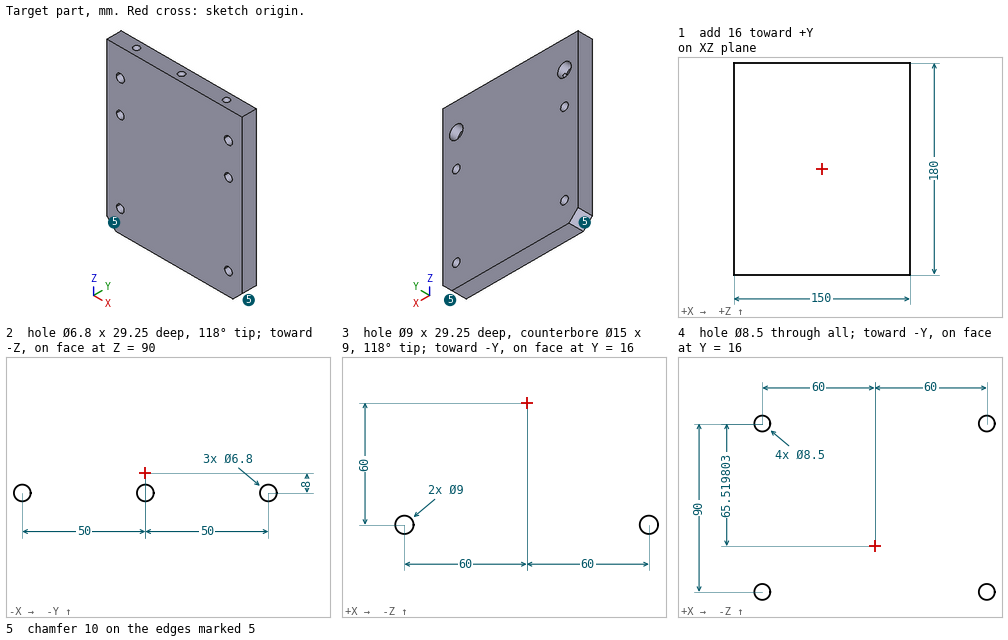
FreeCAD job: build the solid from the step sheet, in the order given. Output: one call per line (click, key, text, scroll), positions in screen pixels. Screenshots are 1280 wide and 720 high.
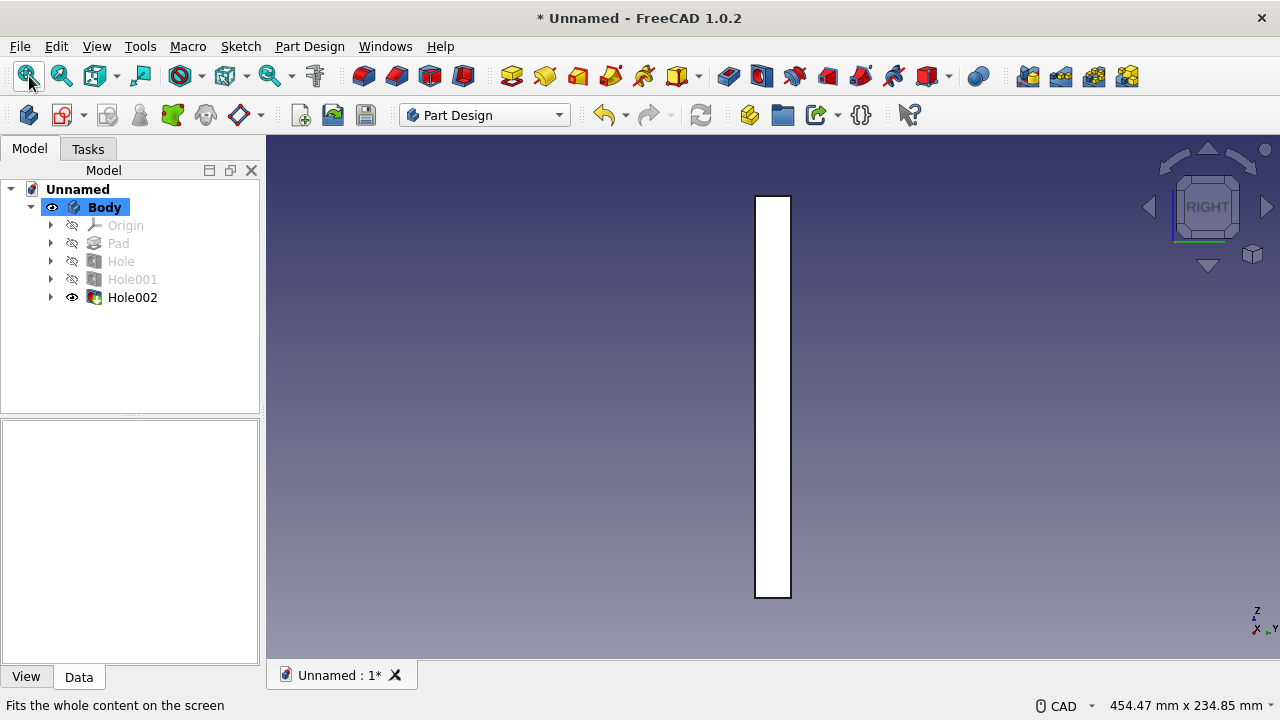
click(773, 597)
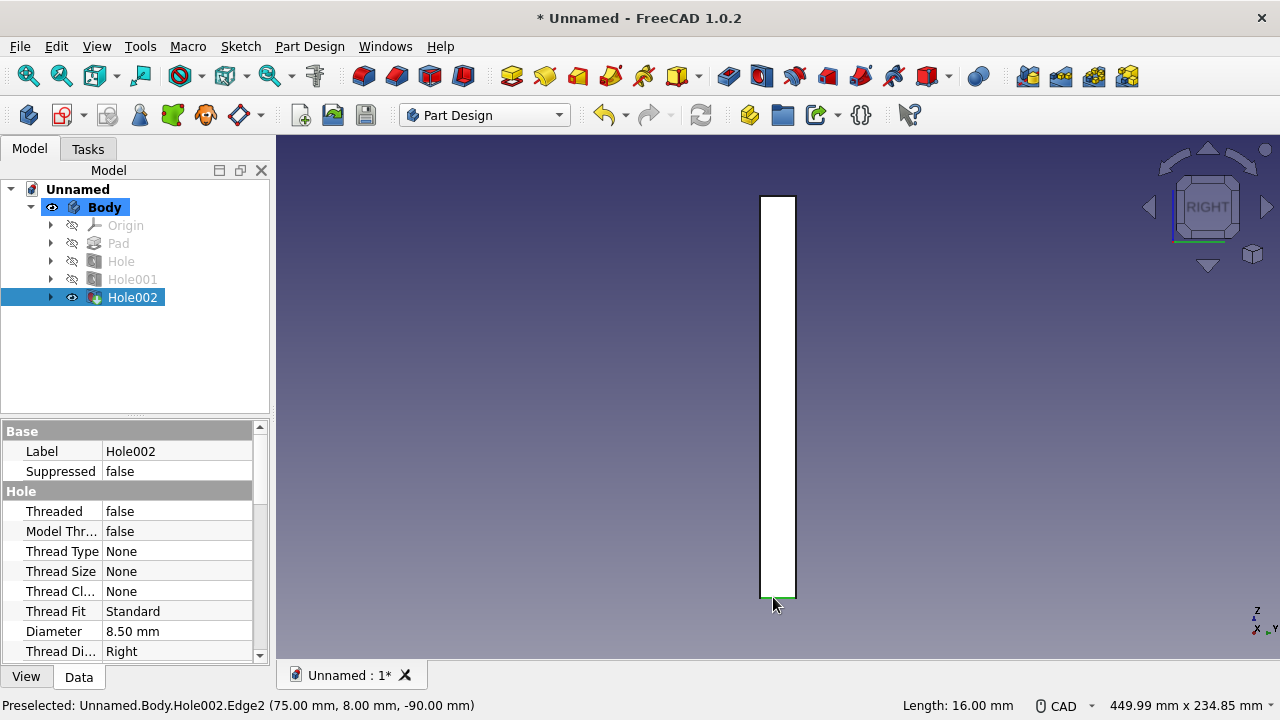
key(5)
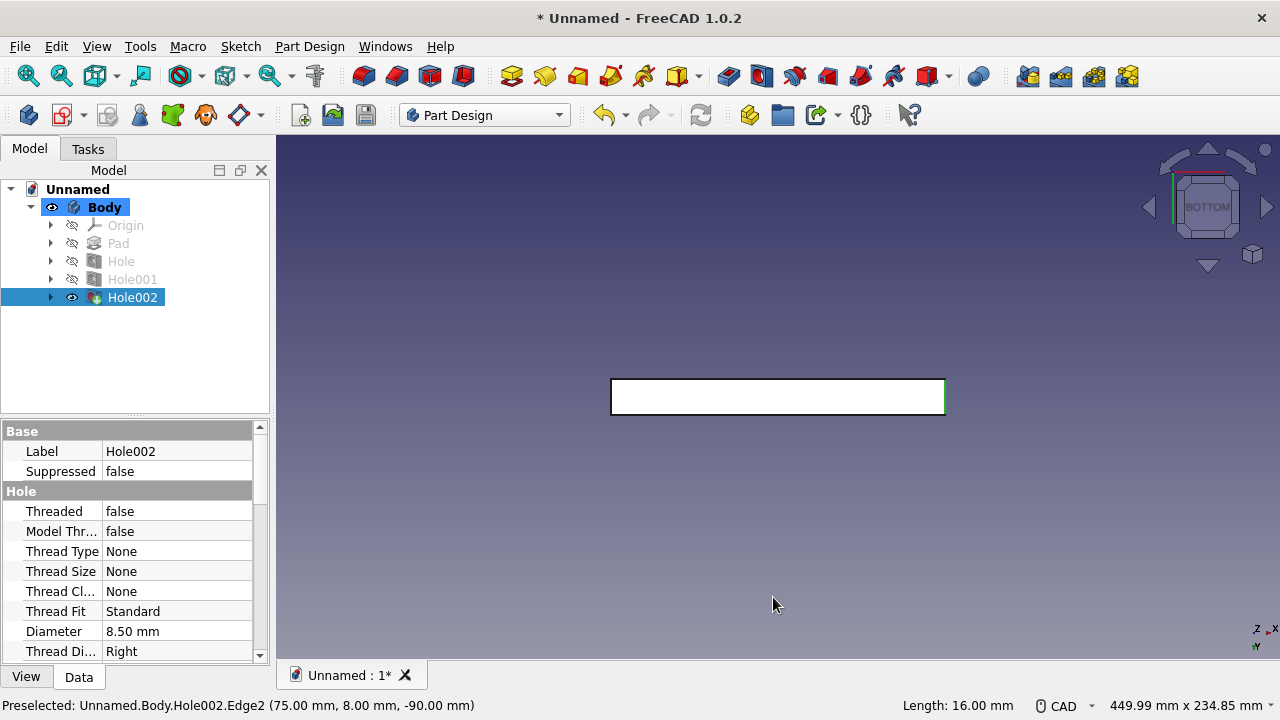
click(29, 76)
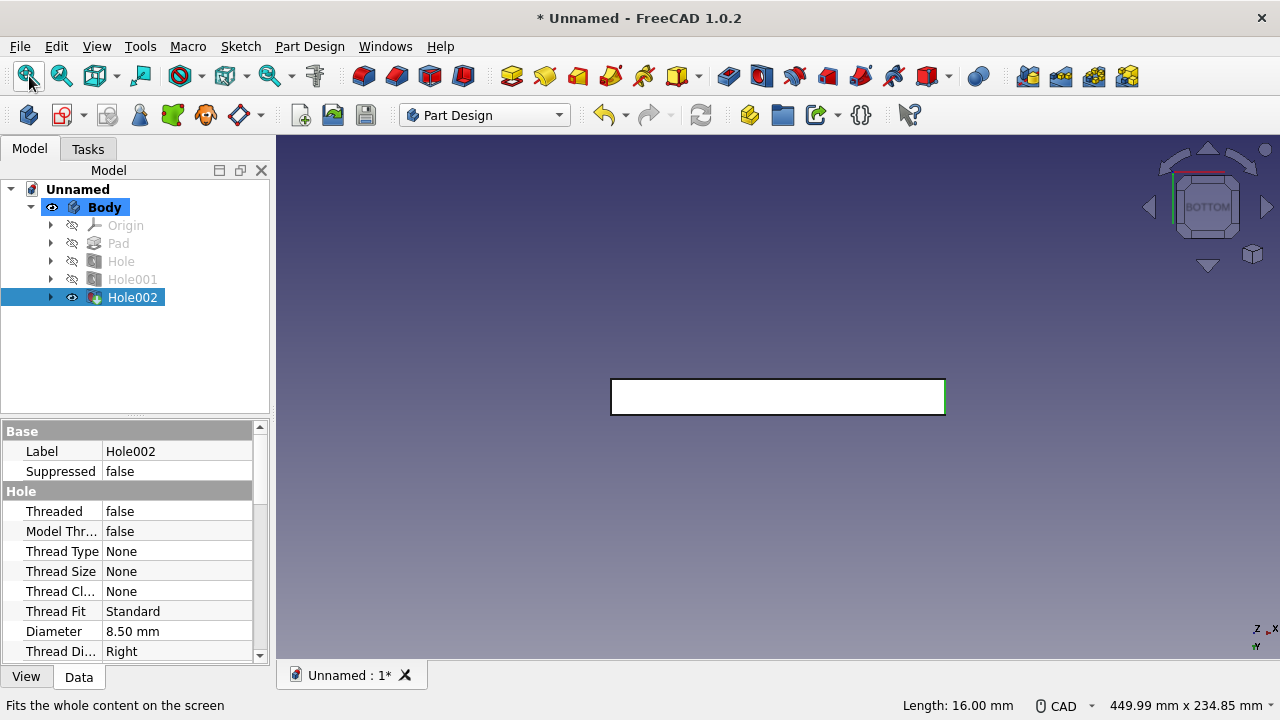
click(611, 396, ctrl)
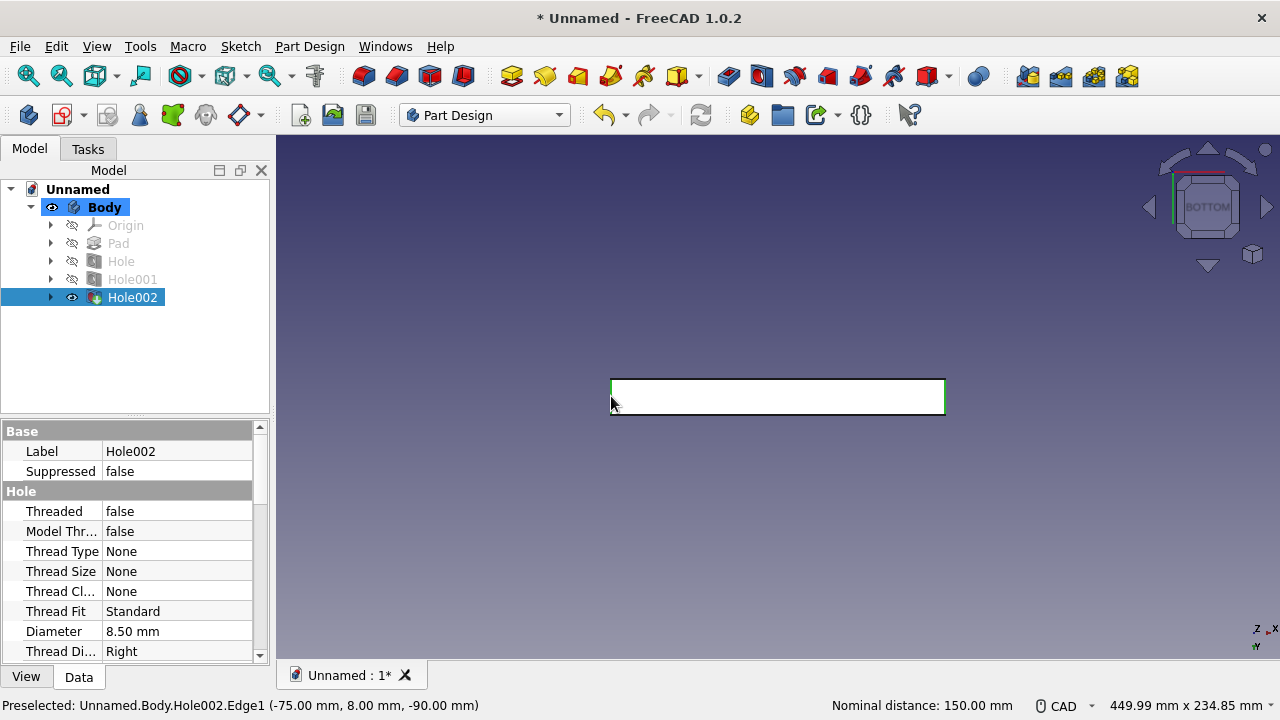
click(397, 76)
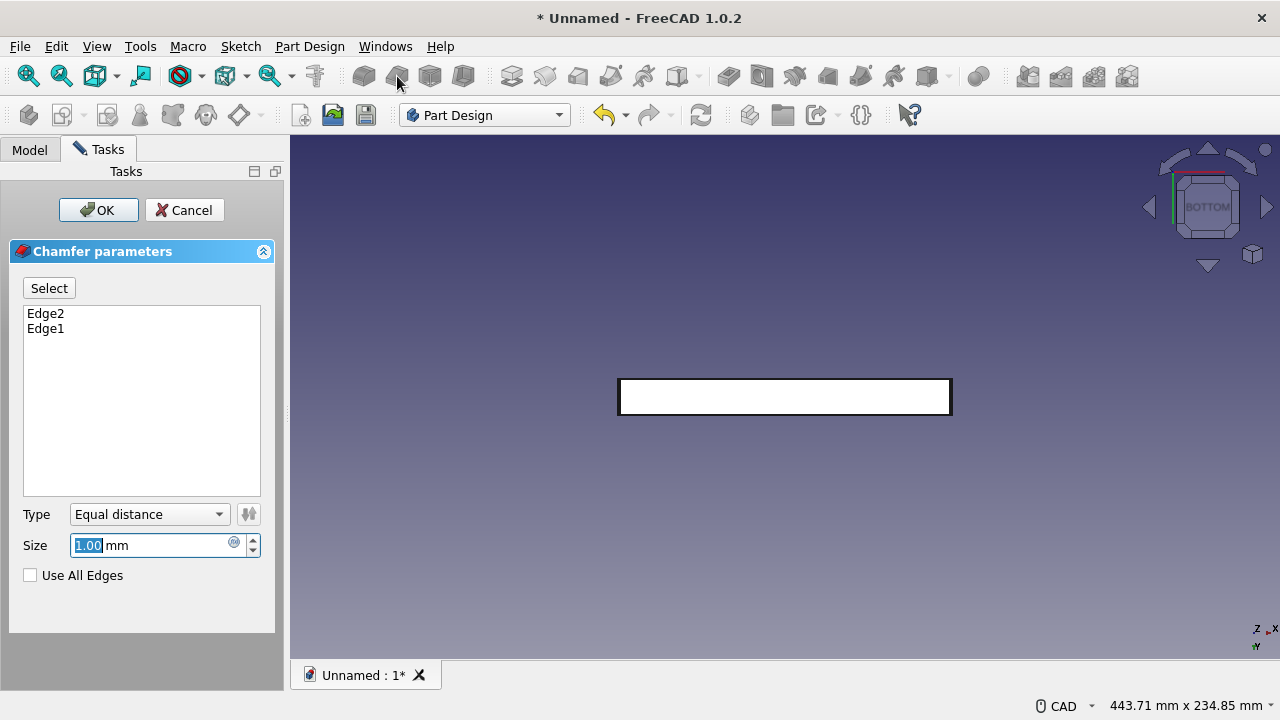
text(10)
key(Tab)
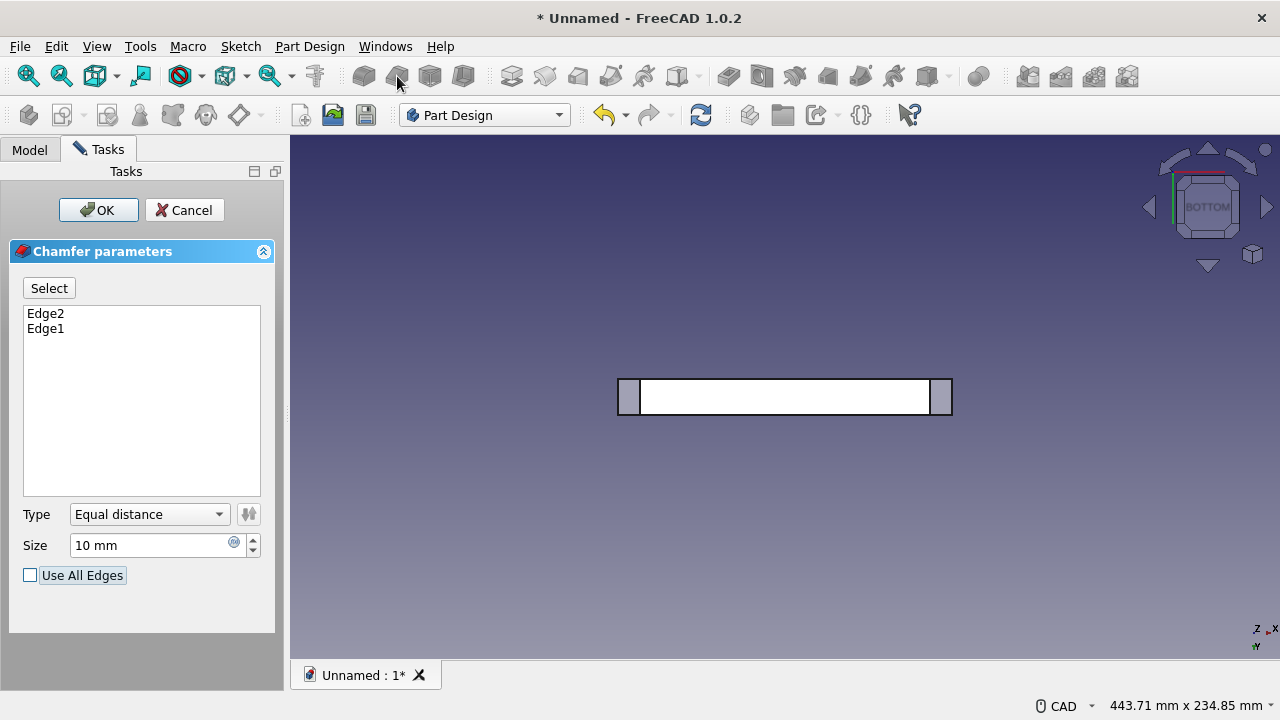
click(99, 210)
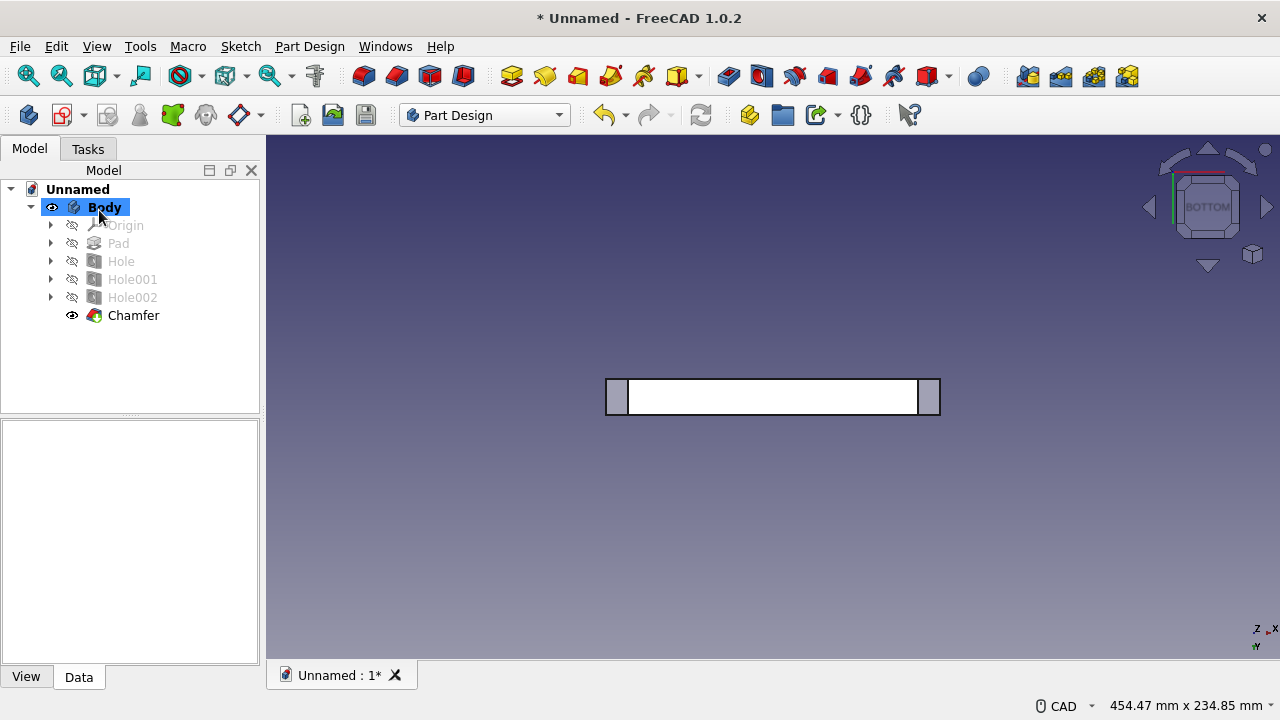
key(0)